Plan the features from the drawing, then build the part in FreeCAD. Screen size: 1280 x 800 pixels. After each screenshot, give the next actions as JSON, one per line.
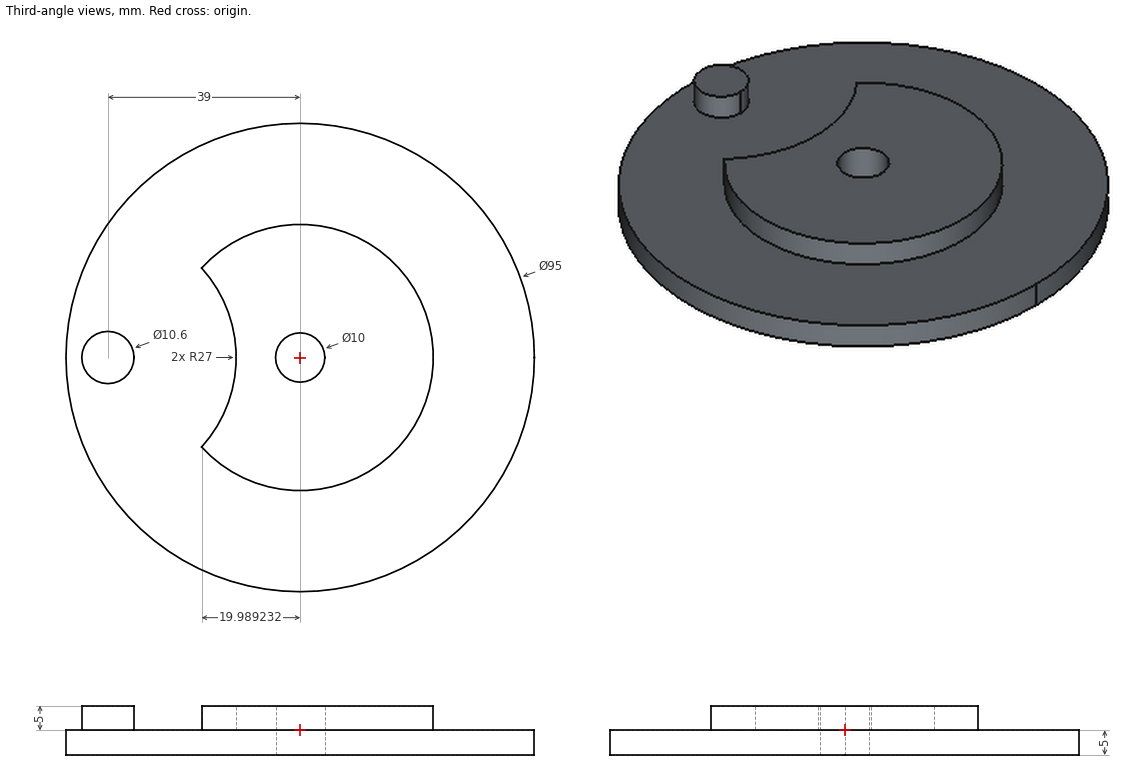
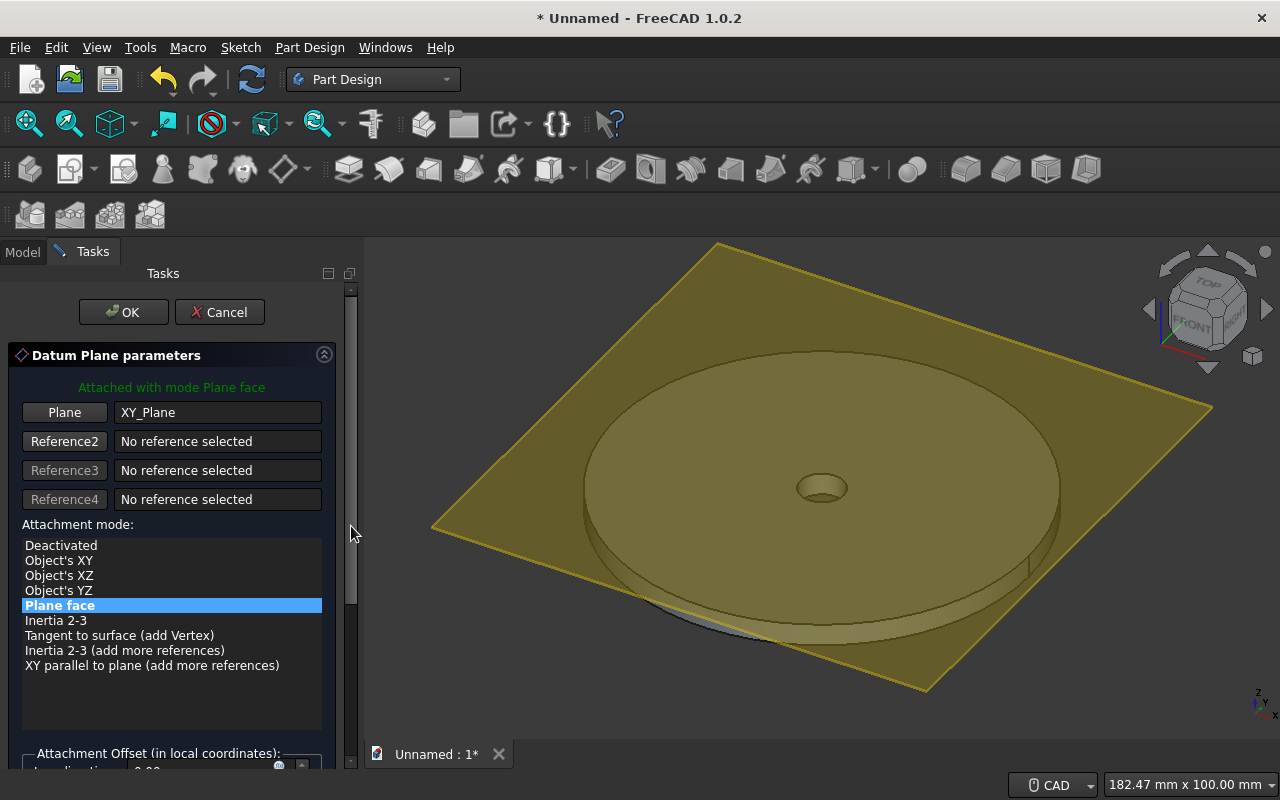
{"action": "left_click", "coordinate": [124, 312]}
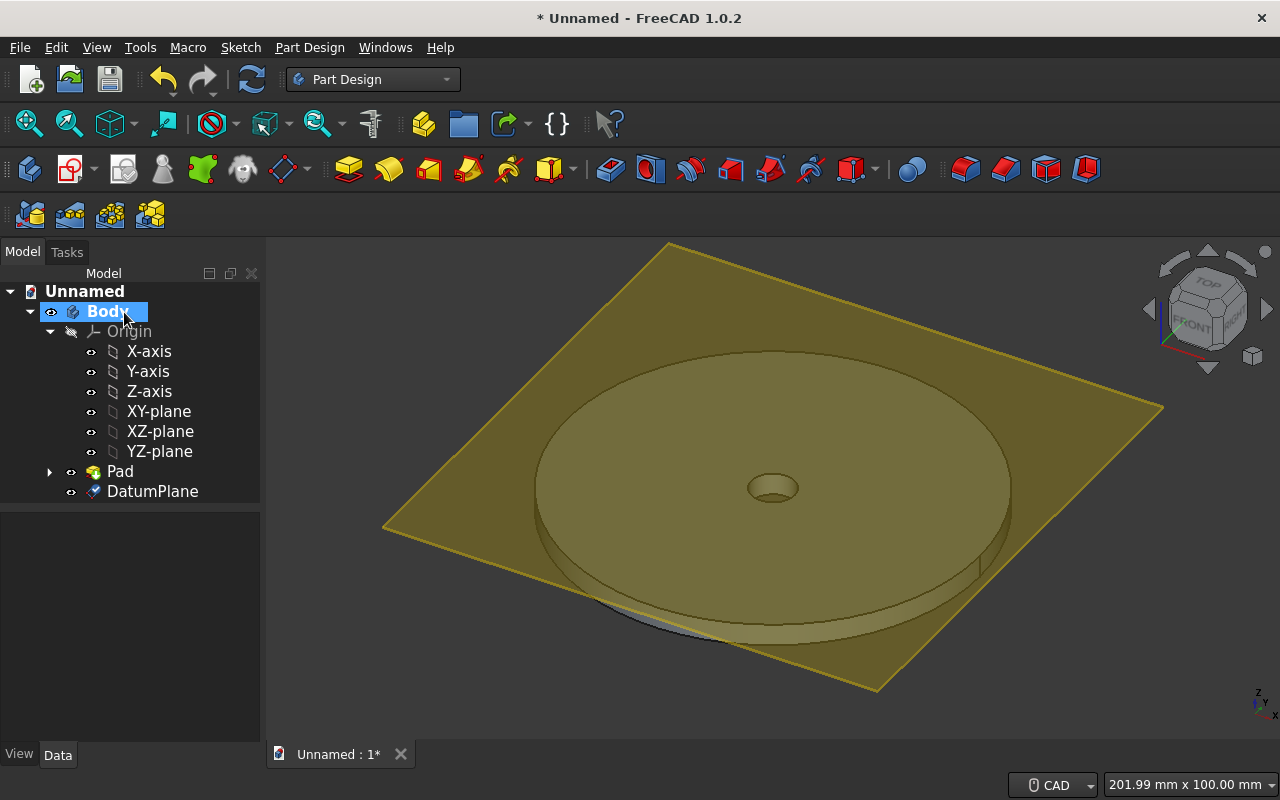
{"action": "left_click", "coordinate": [116, 492]}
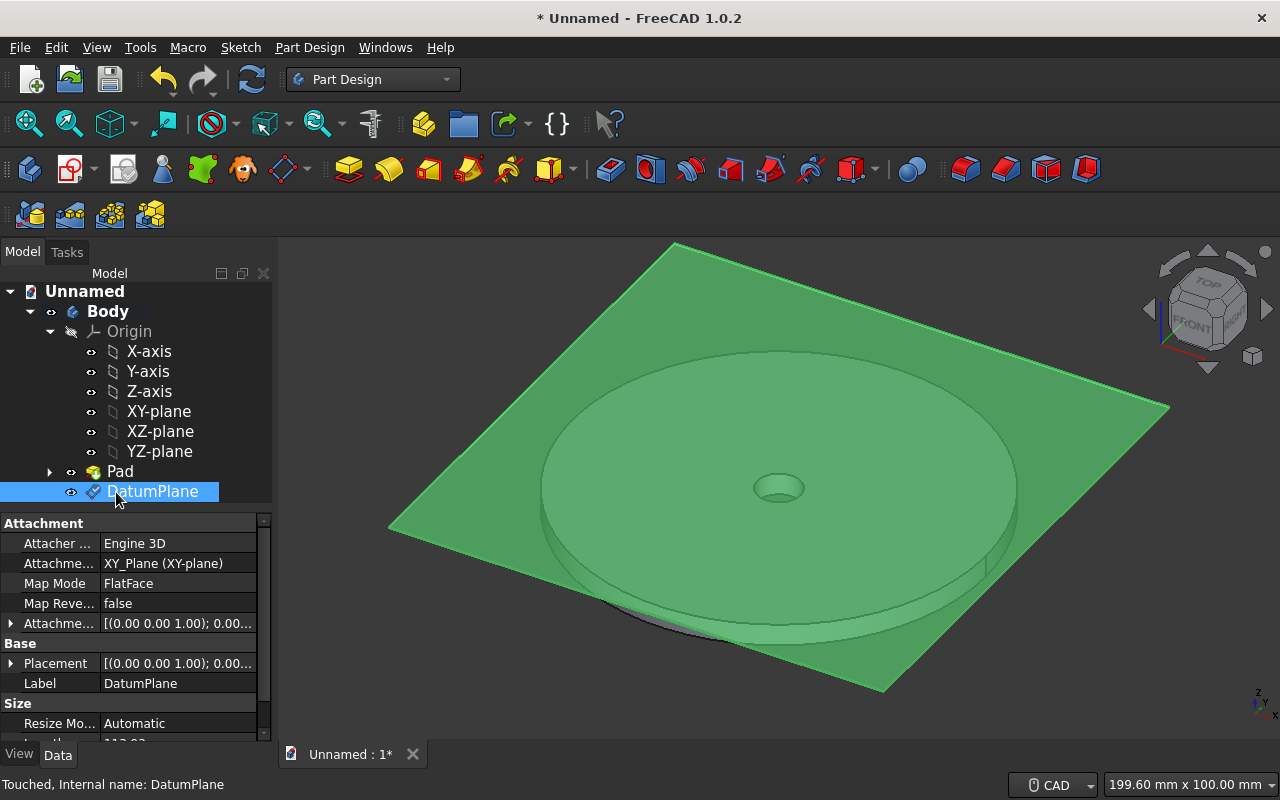
{"action": "left_click", "coordinate": [70, 170]}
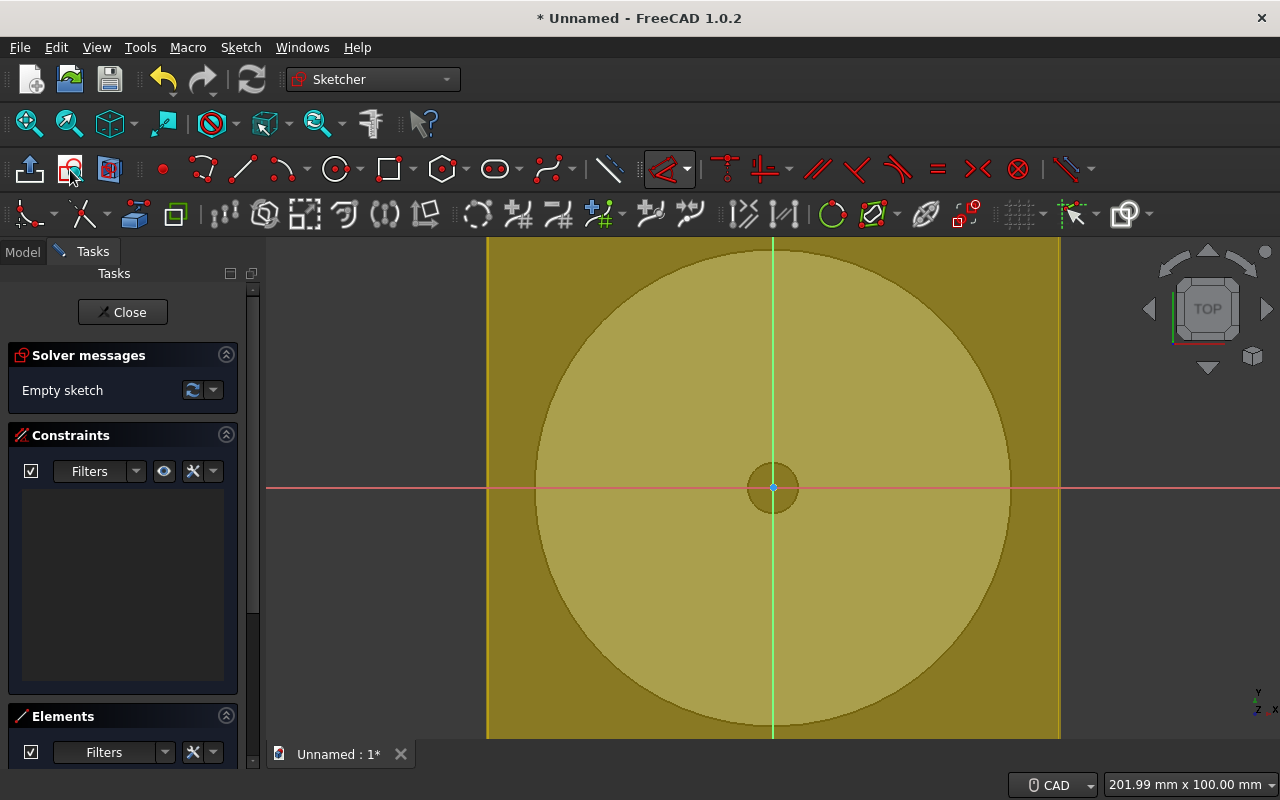
{"action": "scroll", "coordinate": [781, 488], "scroll_direction": "up", "scroll_amount": 2}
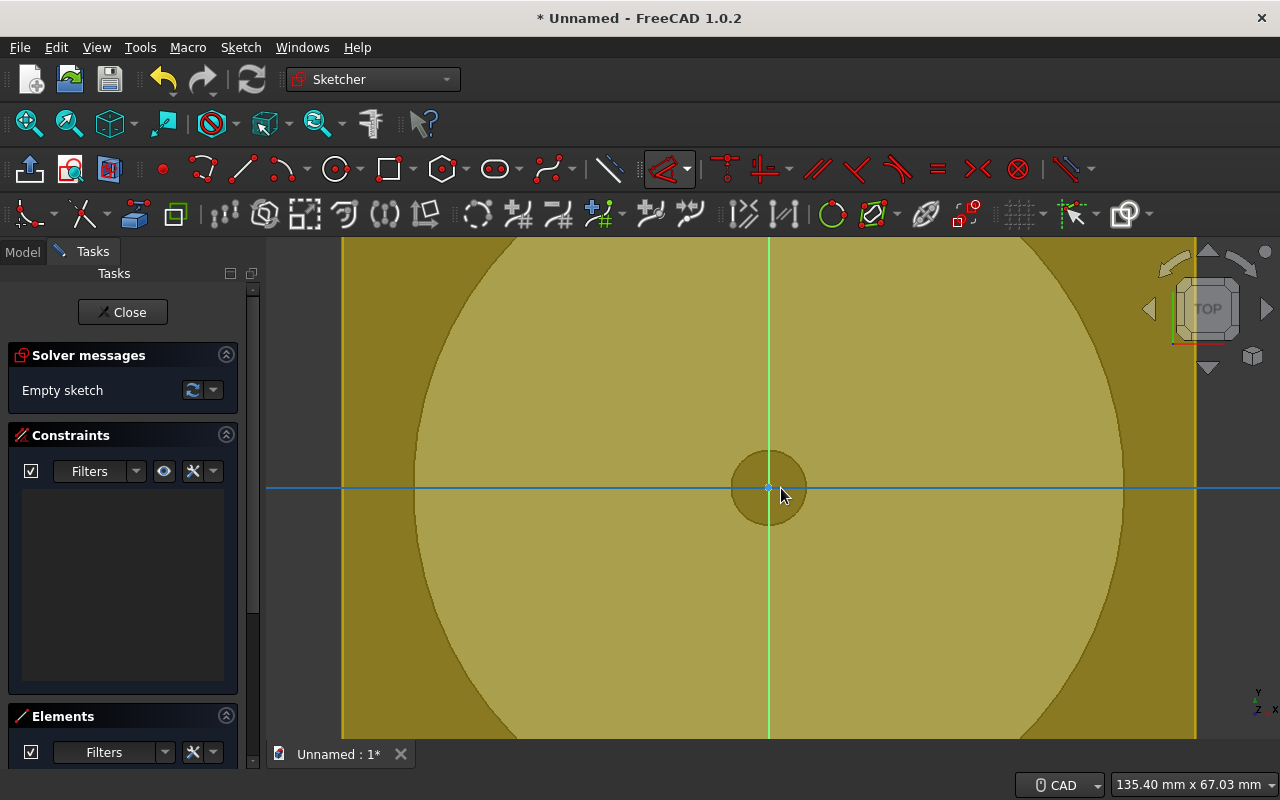
{"action": "key", "text": "g 3 a"}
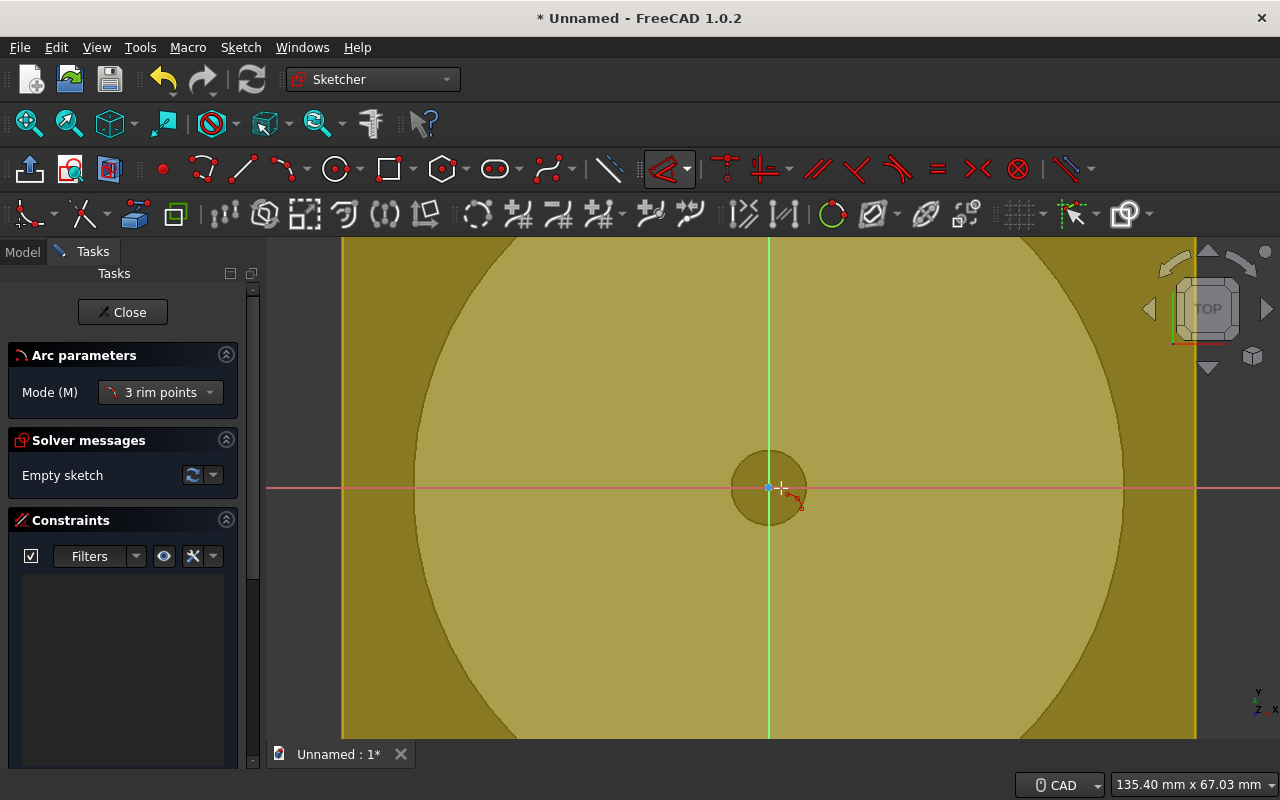
{"action": "left_click", "coordinate": [619, 624]}
{"action": "left_click", "coordinate": [619, 352]}
{"action": "left_click", "coordinate": [669, 517]}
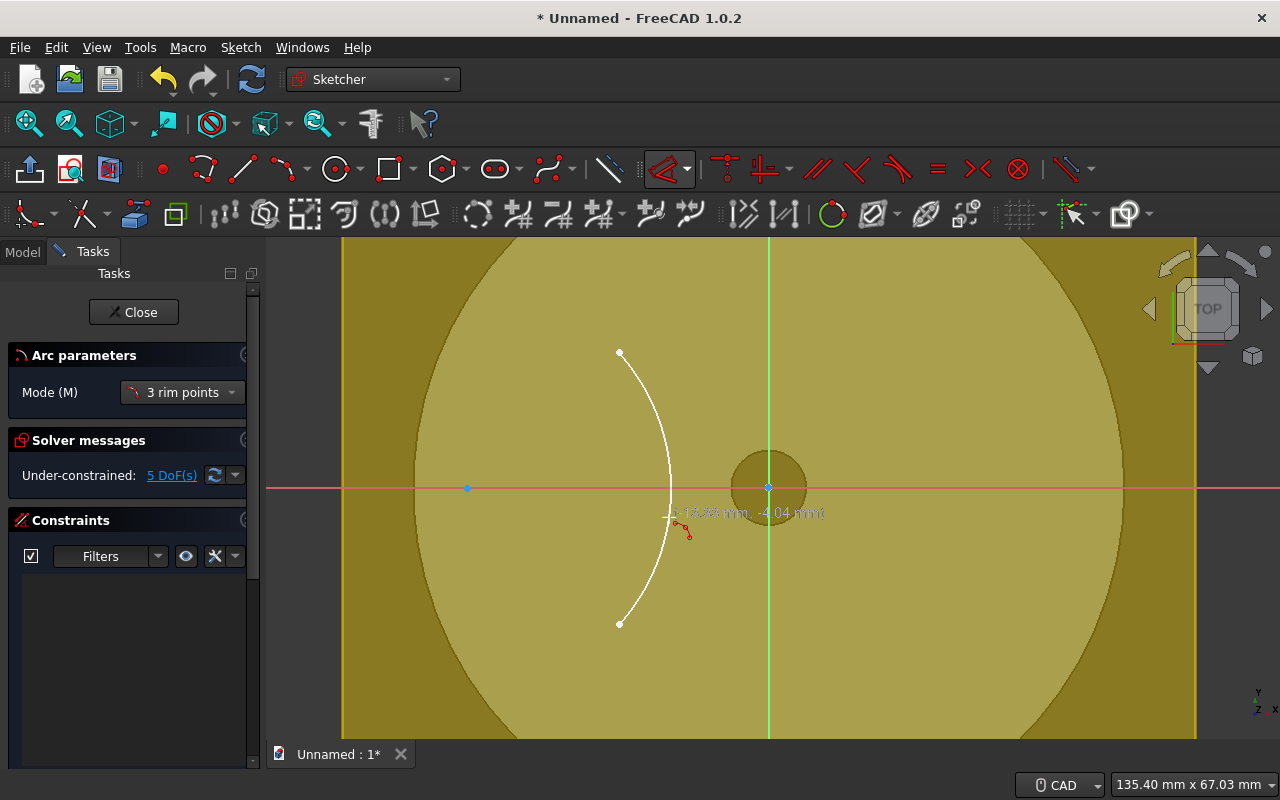
{"action": "left_click", "coordinate": [619, 353]}
{"action": "left_click", "coordinate": [619, 625]}
{"action": "left_click", "coordinate": [948, 581]}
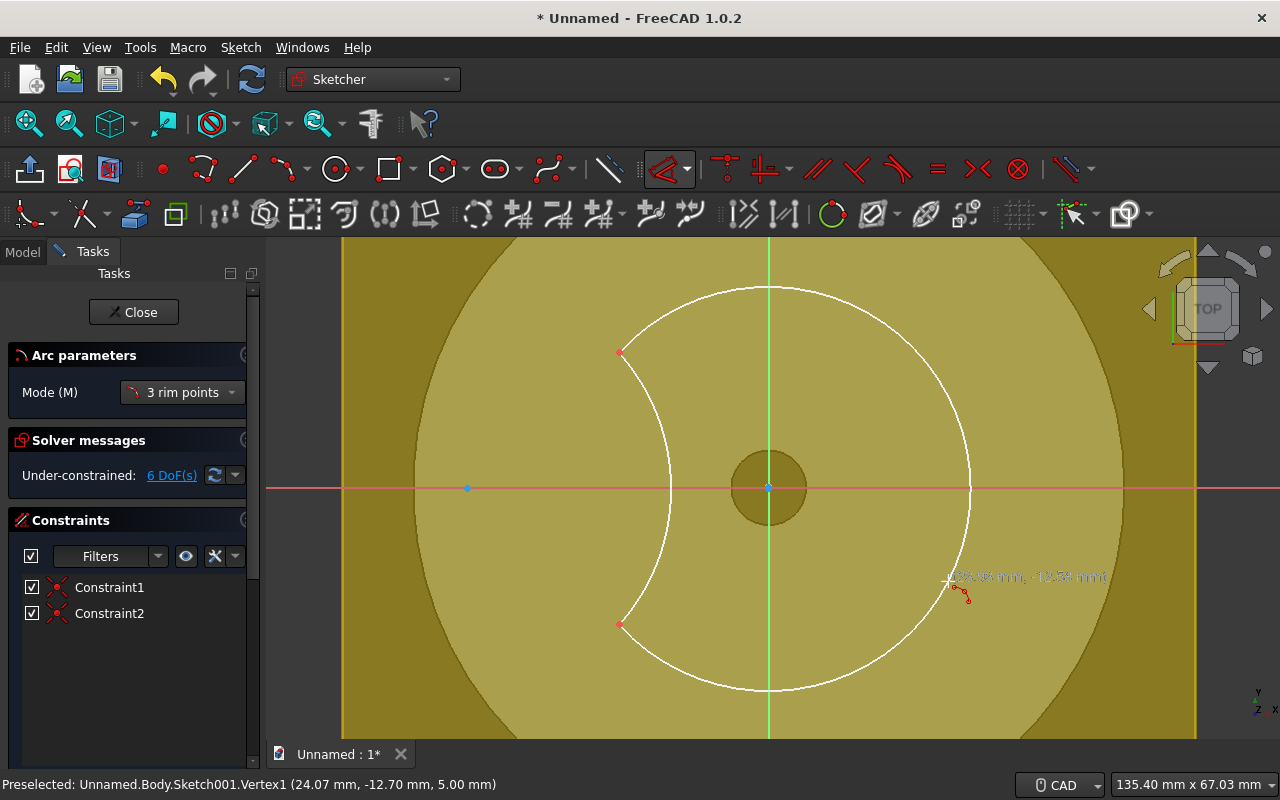
{"action": "key", "text": "g c"}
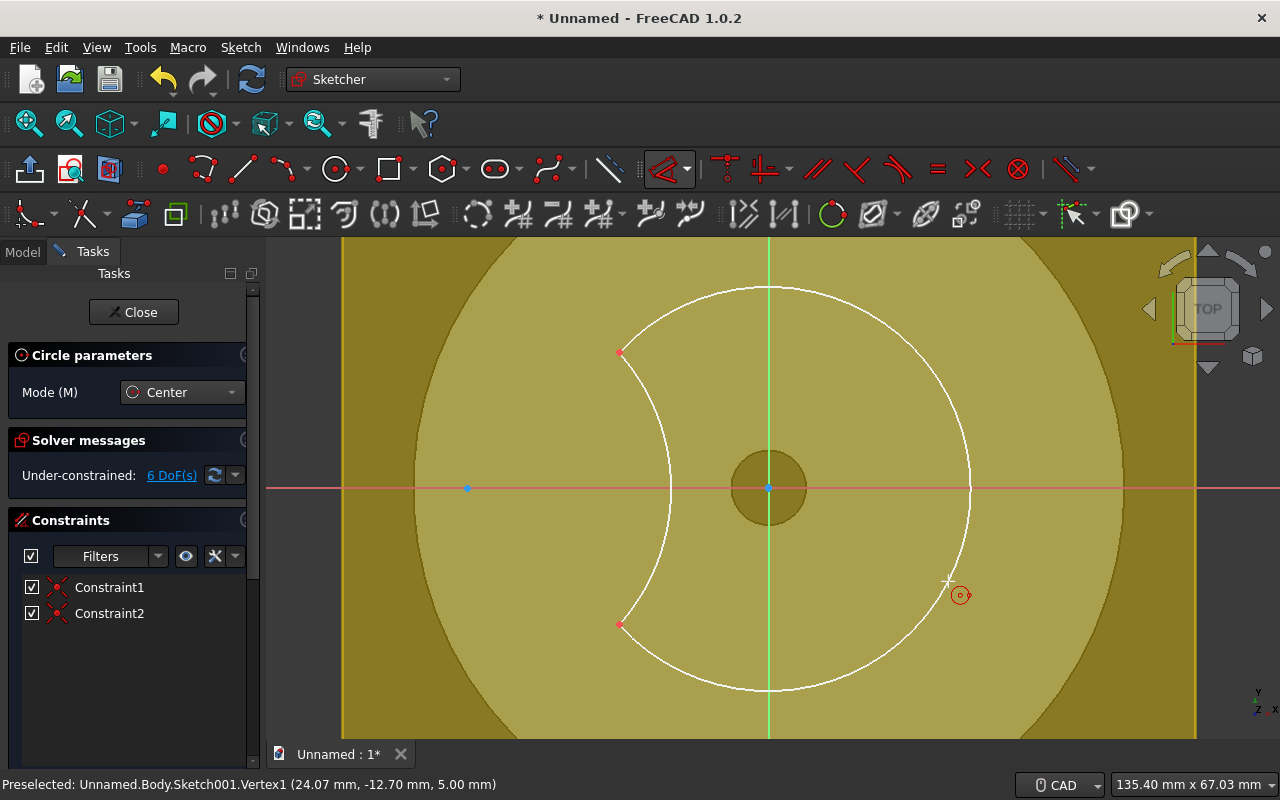
{"action": "scroll", "coordinate": [477, 488], "scroll_direction": "up", "scroll_amount": 4}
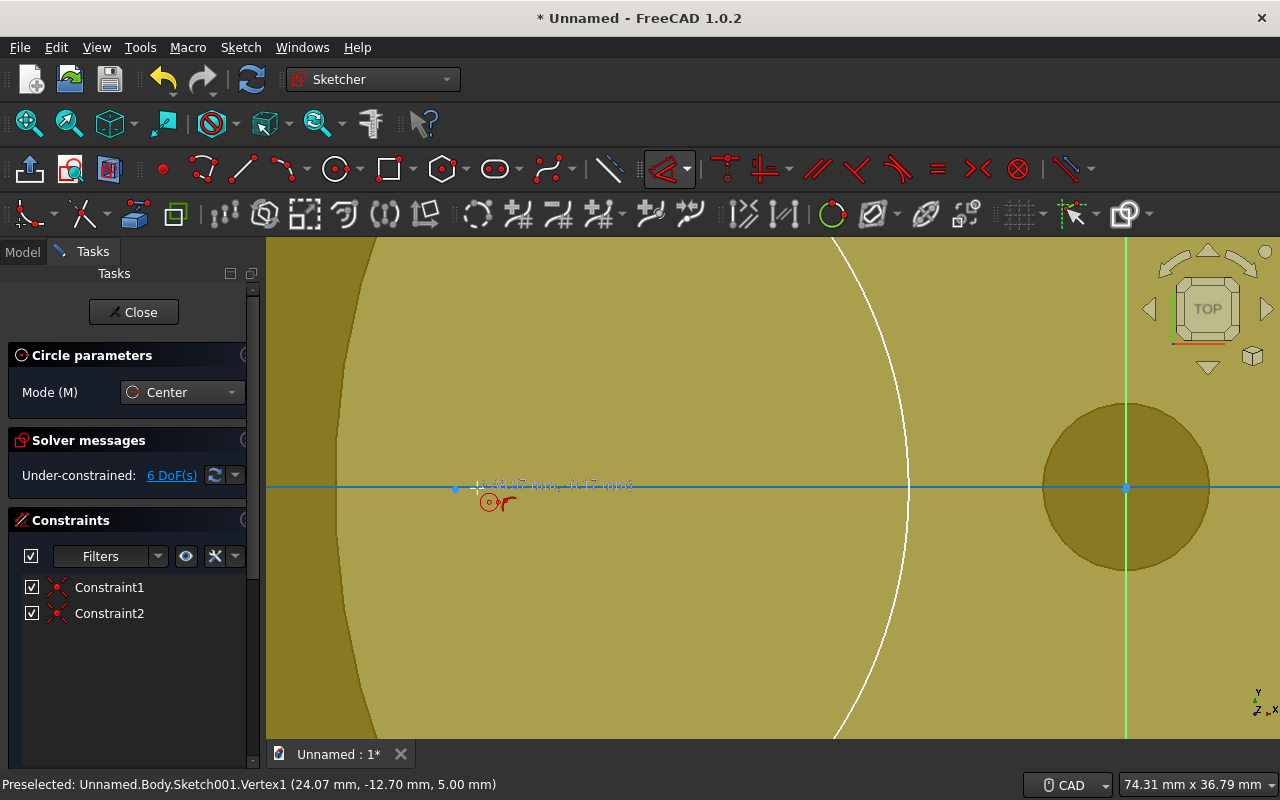
{"action": "left_click", "coordinate": [476, 487]}
{"action": "left_click", "coordinate": [539, 424]}